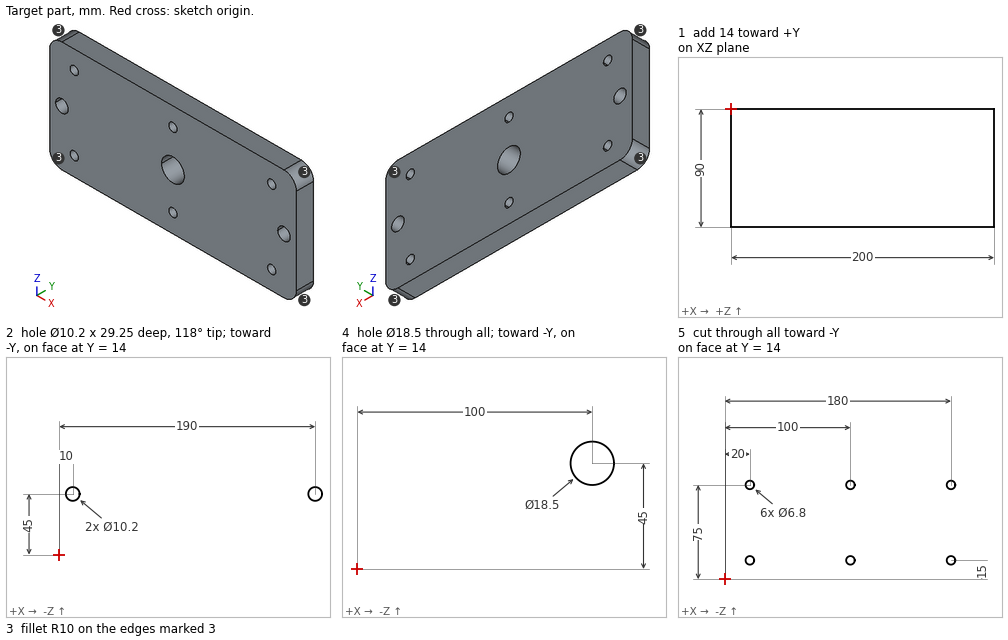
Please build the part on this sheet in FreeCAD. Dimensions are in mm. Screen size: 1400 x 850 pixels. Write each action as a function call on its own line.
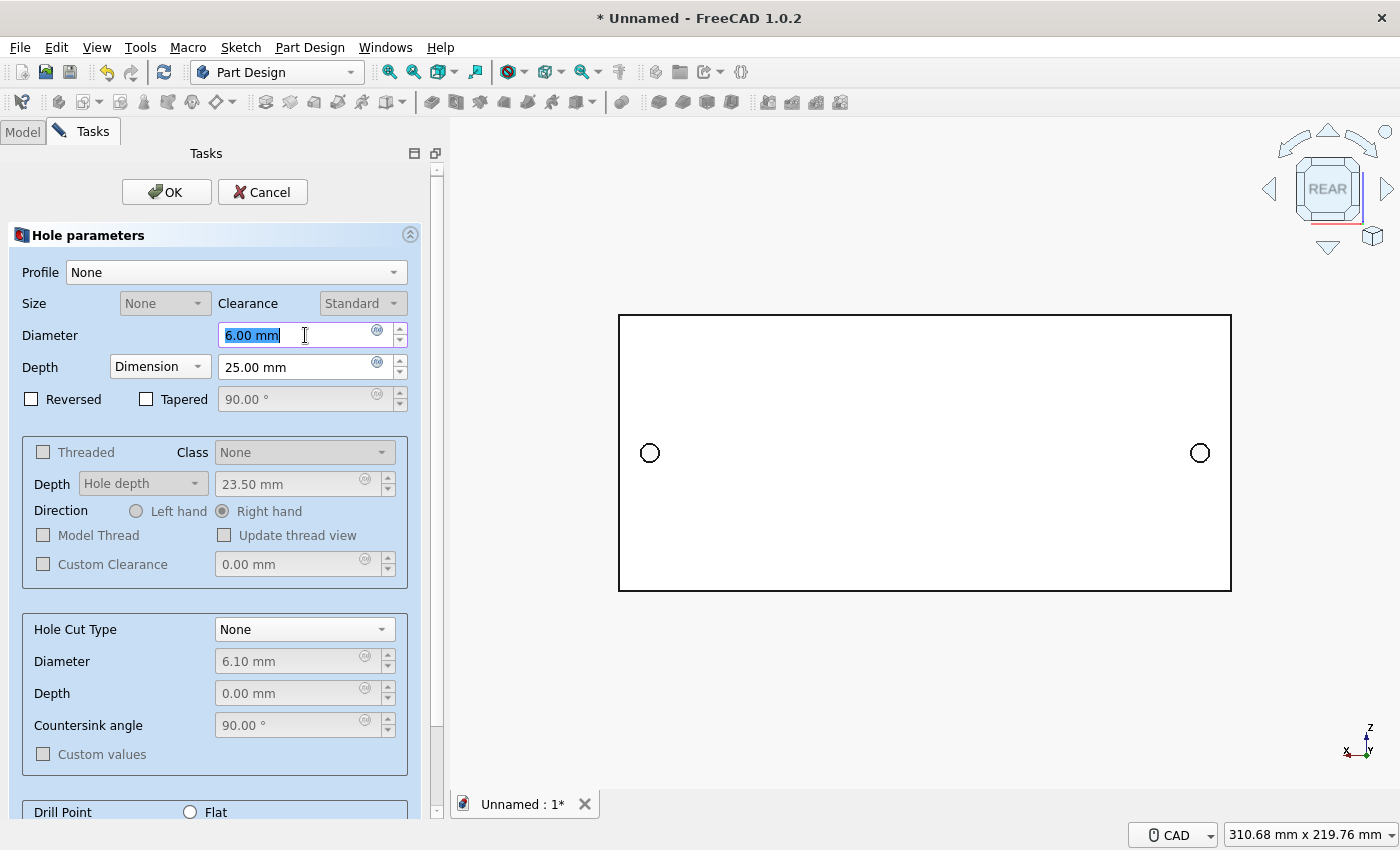
text(10.2)
key(Tab)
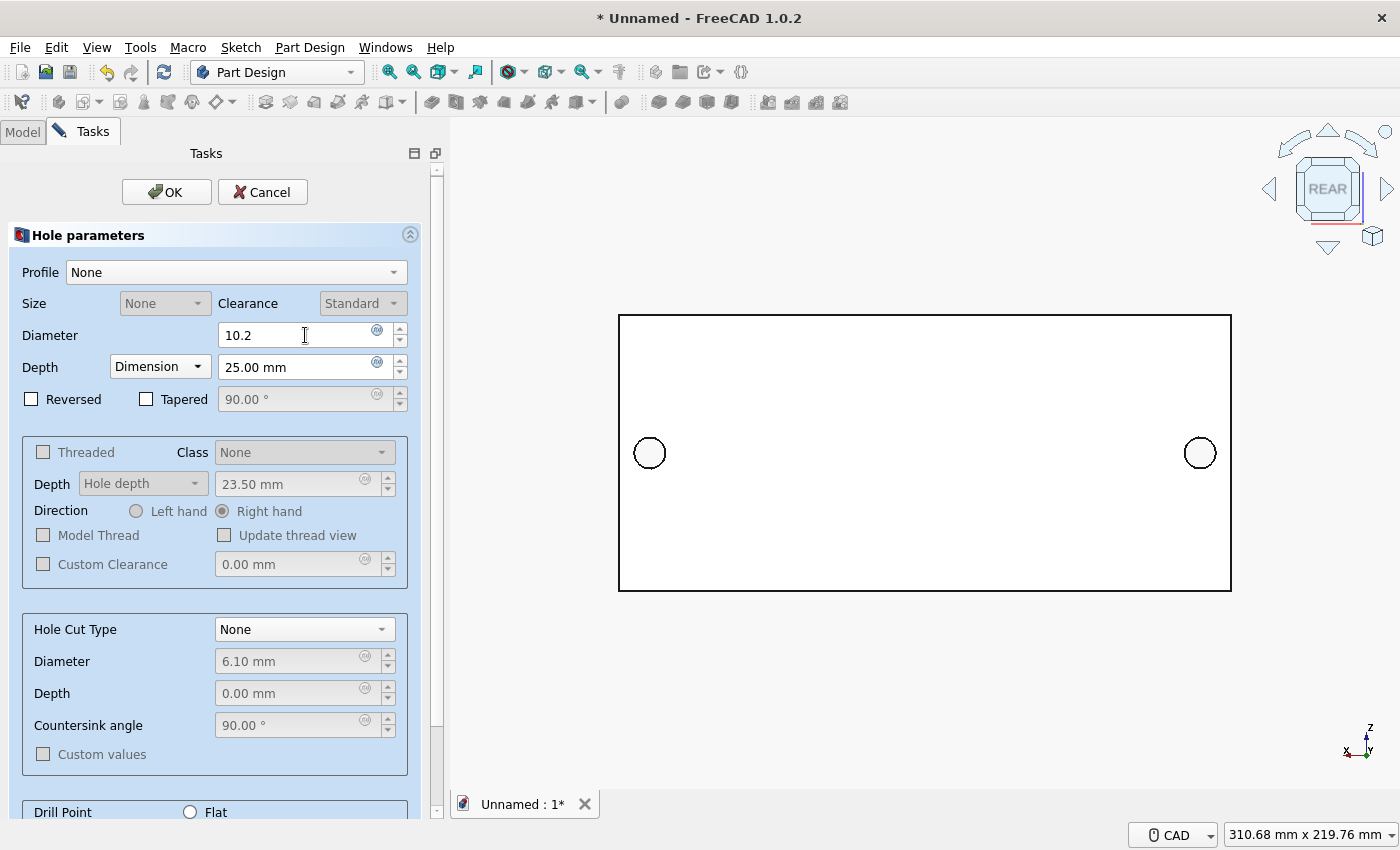
triple_click(305, 367)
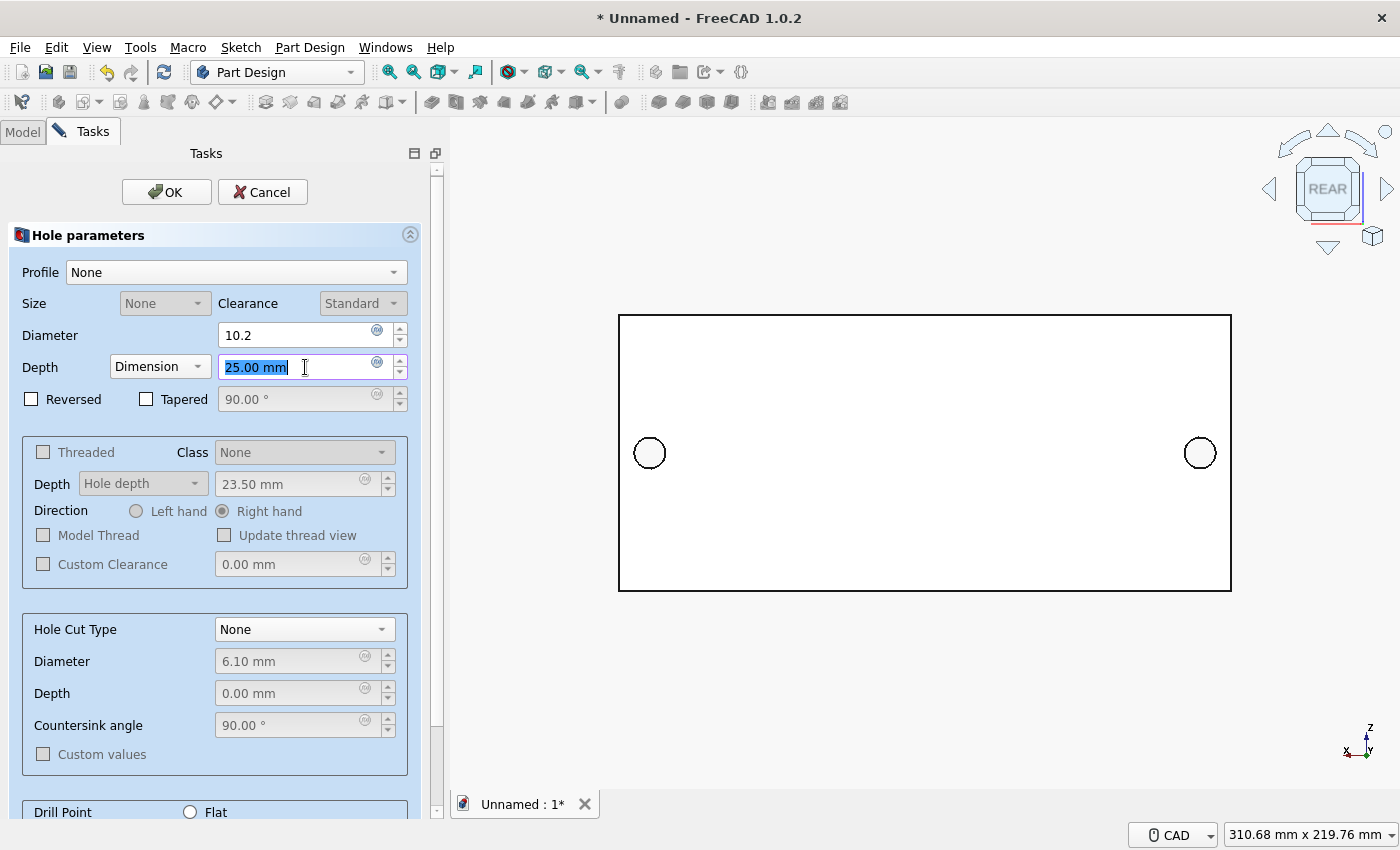
text(29.25)
key(Tab)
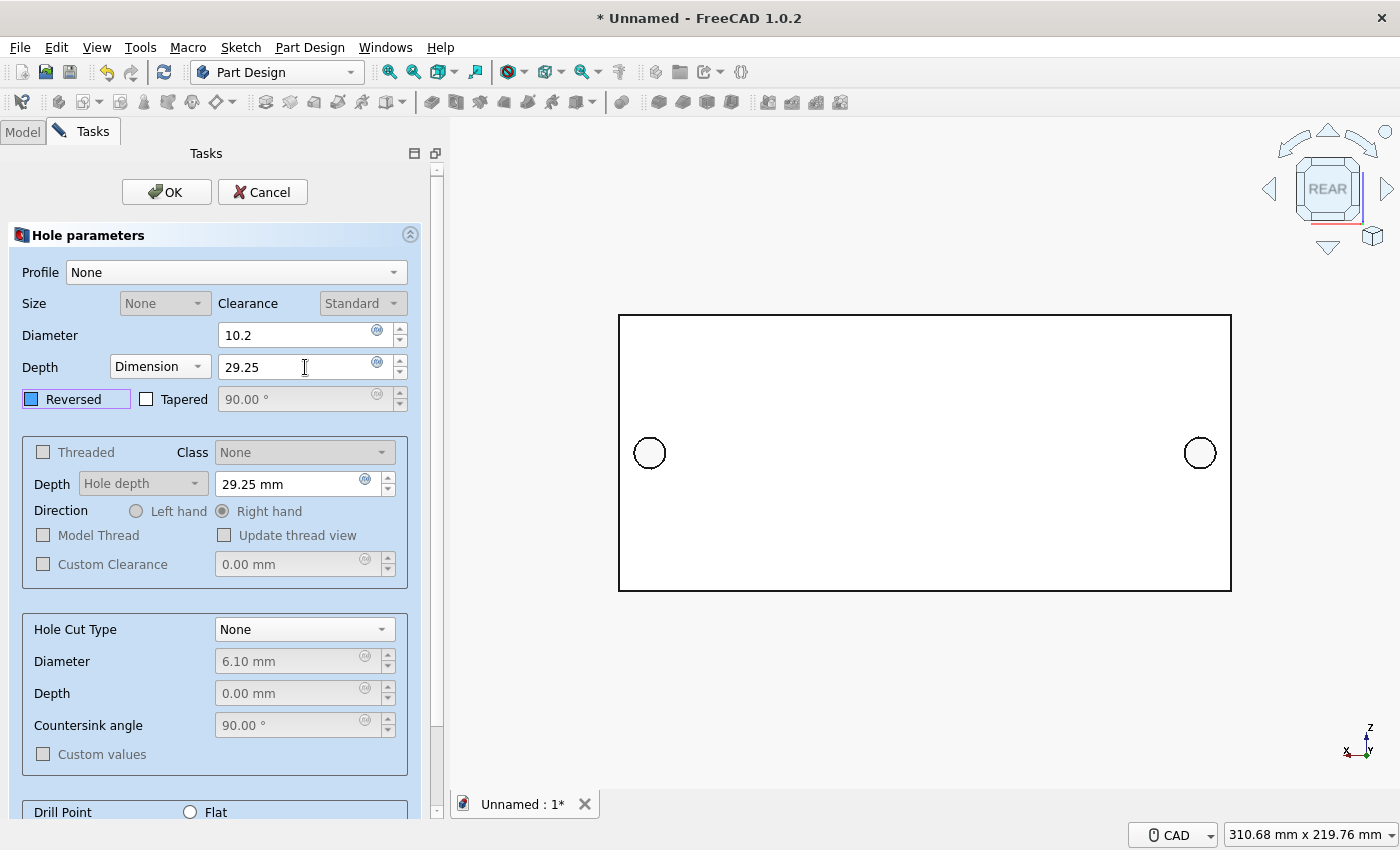
click(167, 192)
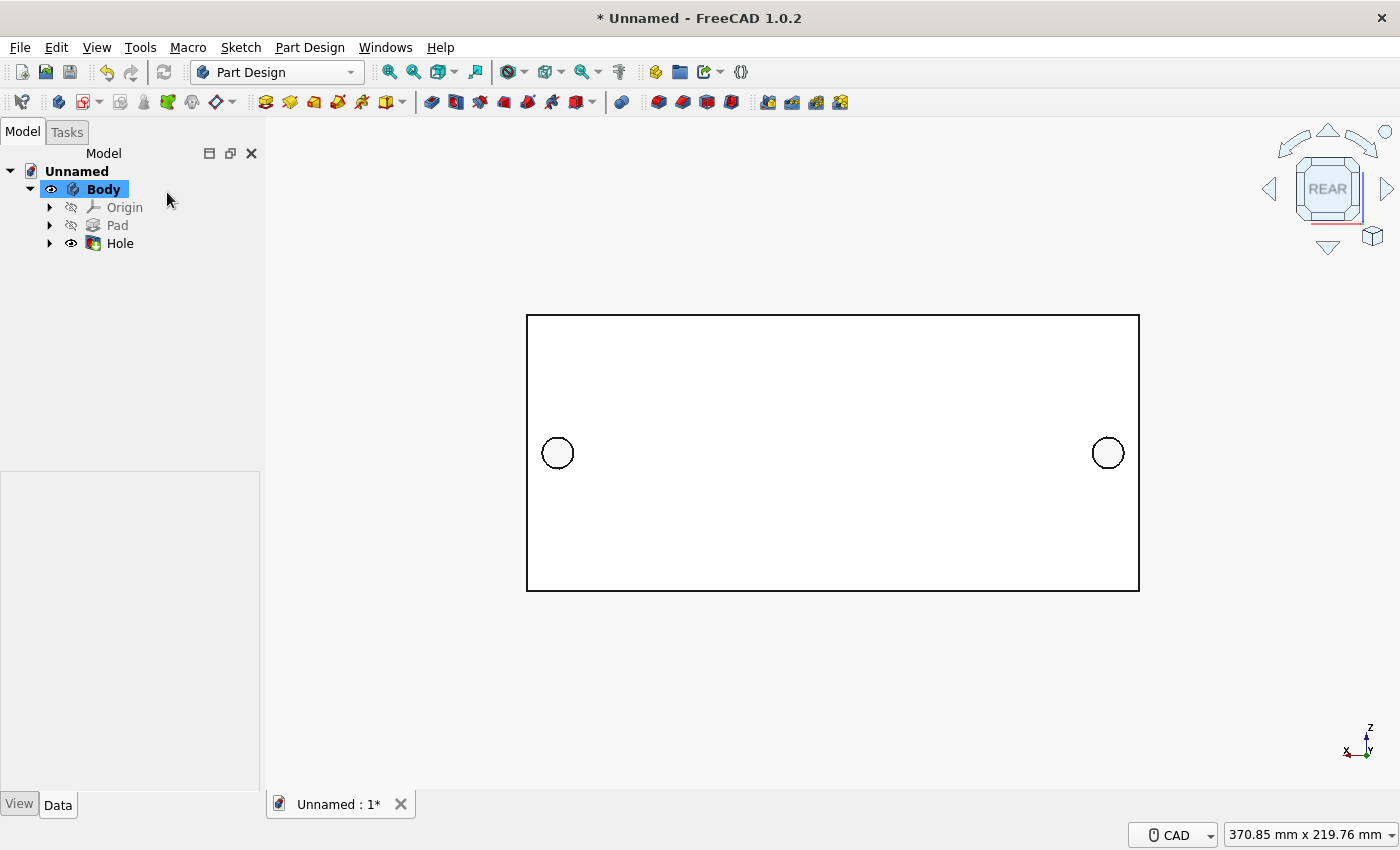
key(0)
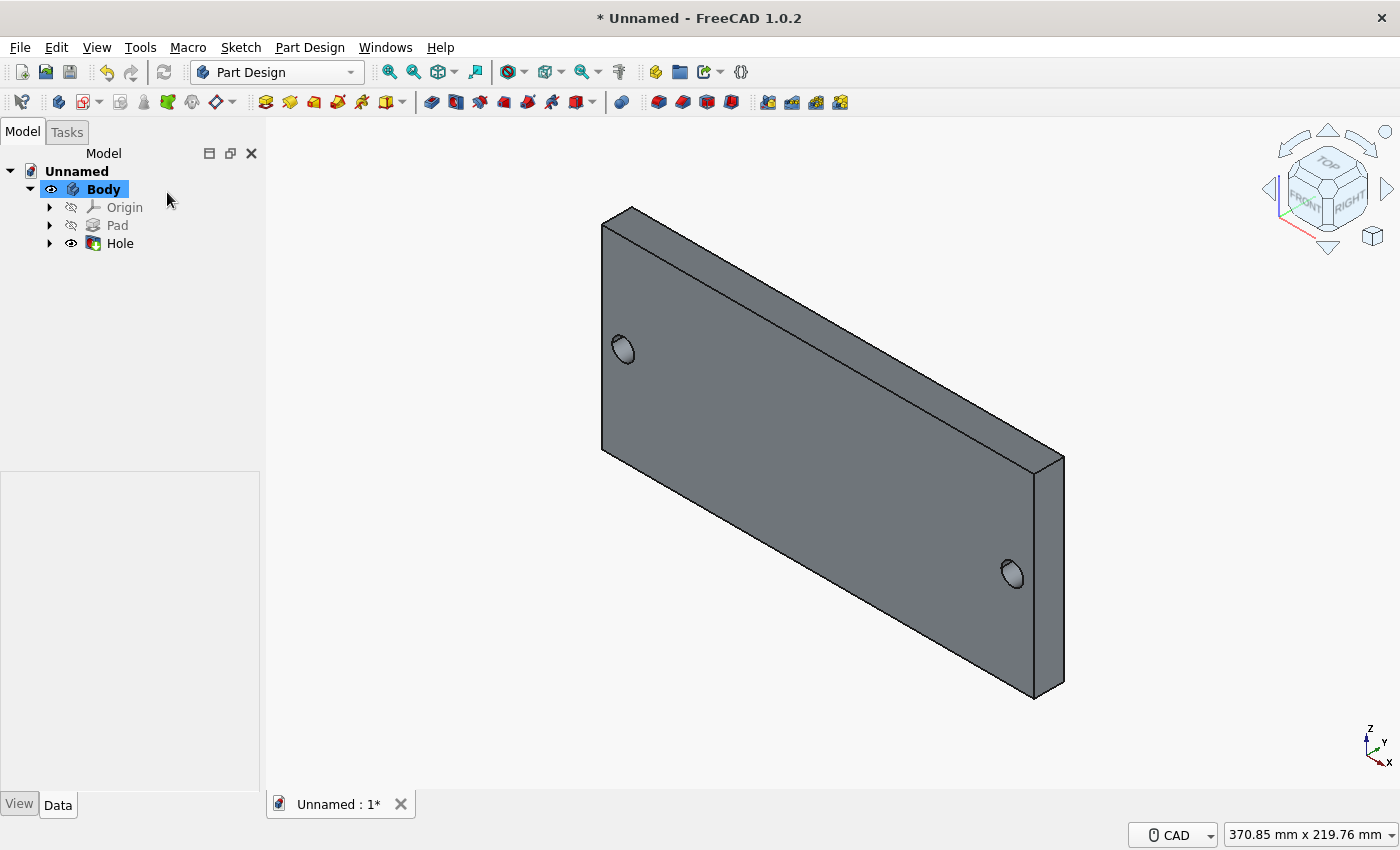
click(1049, 464)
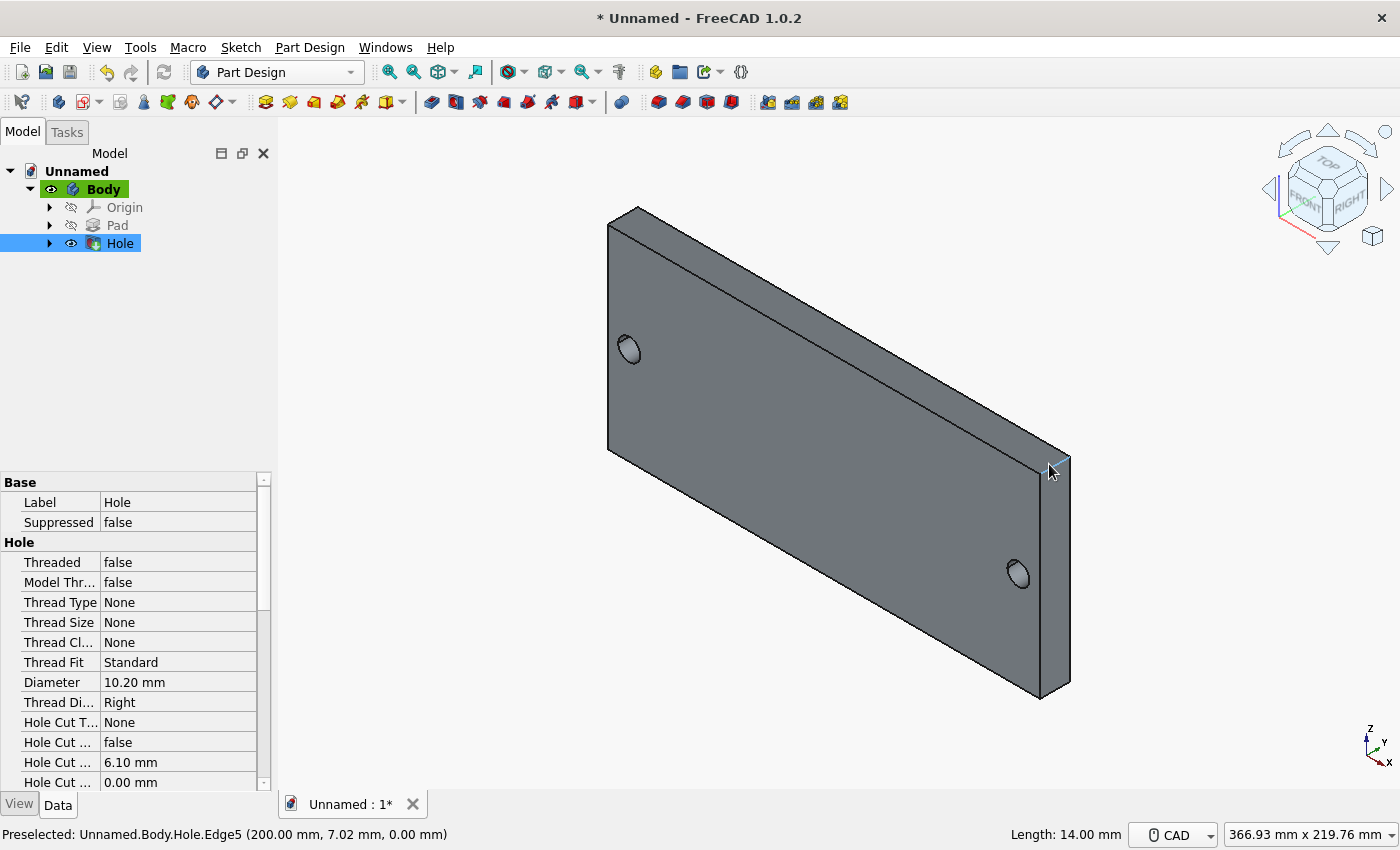
key(2)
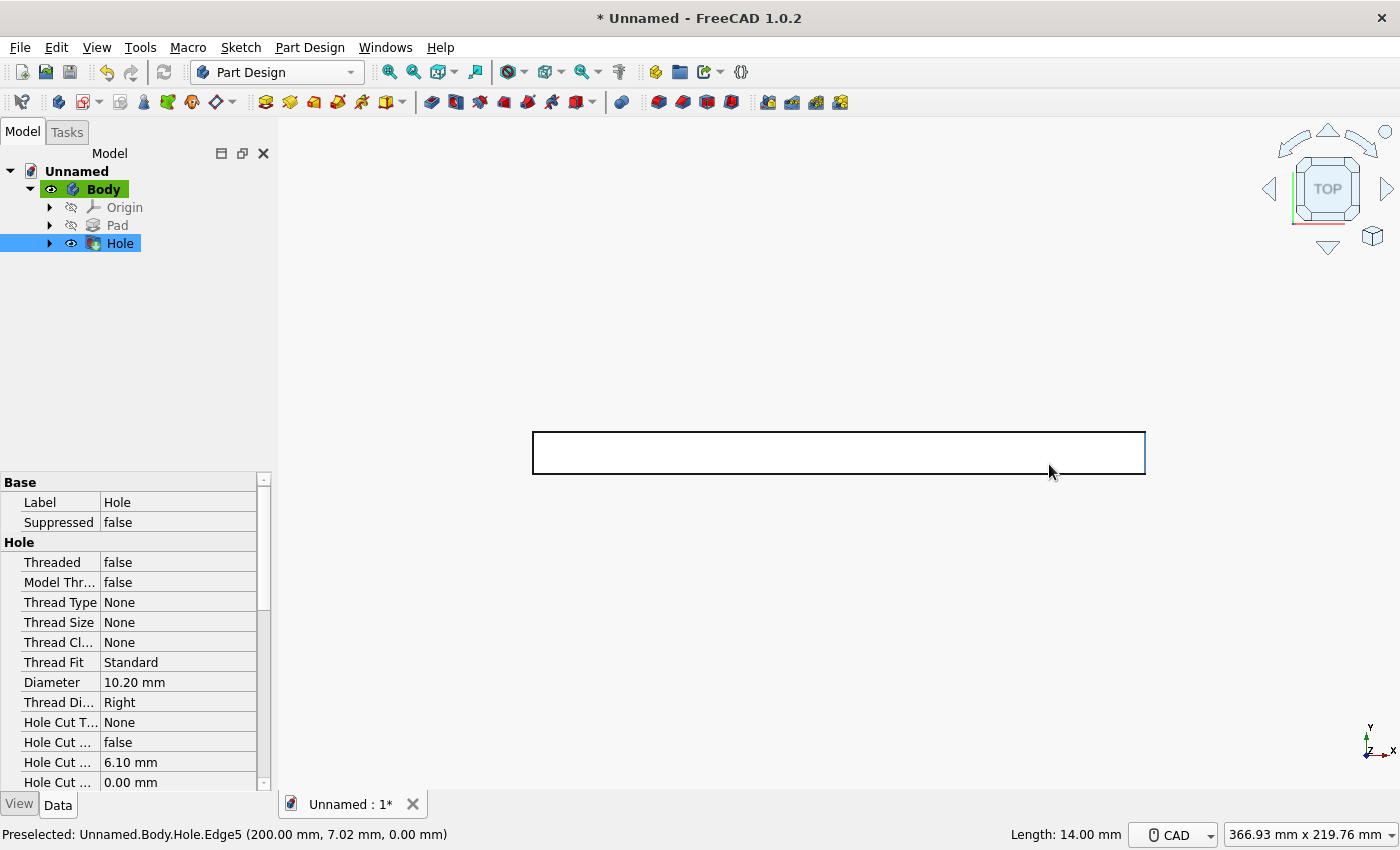
click(533, 456, ctrl)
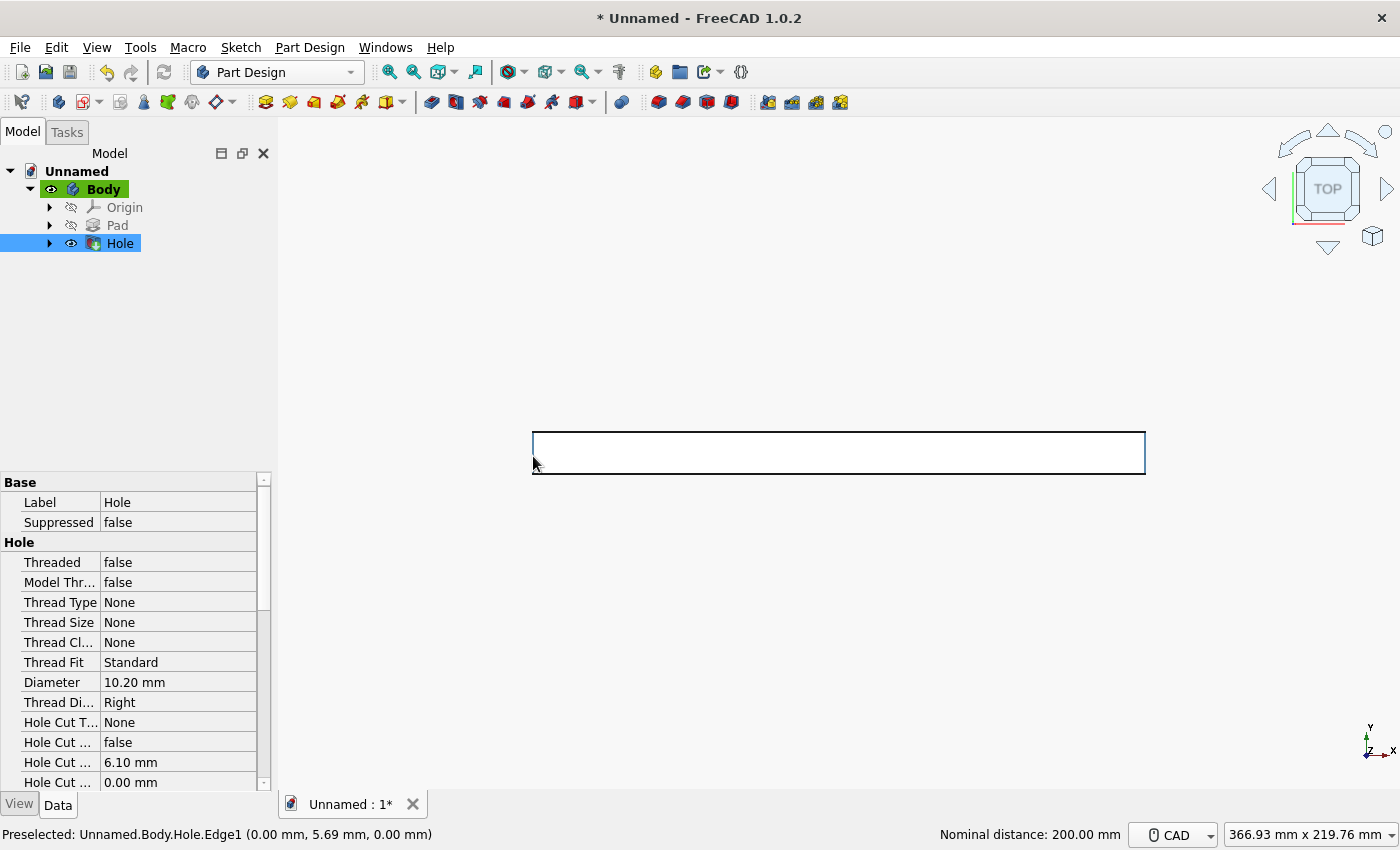
key(1)